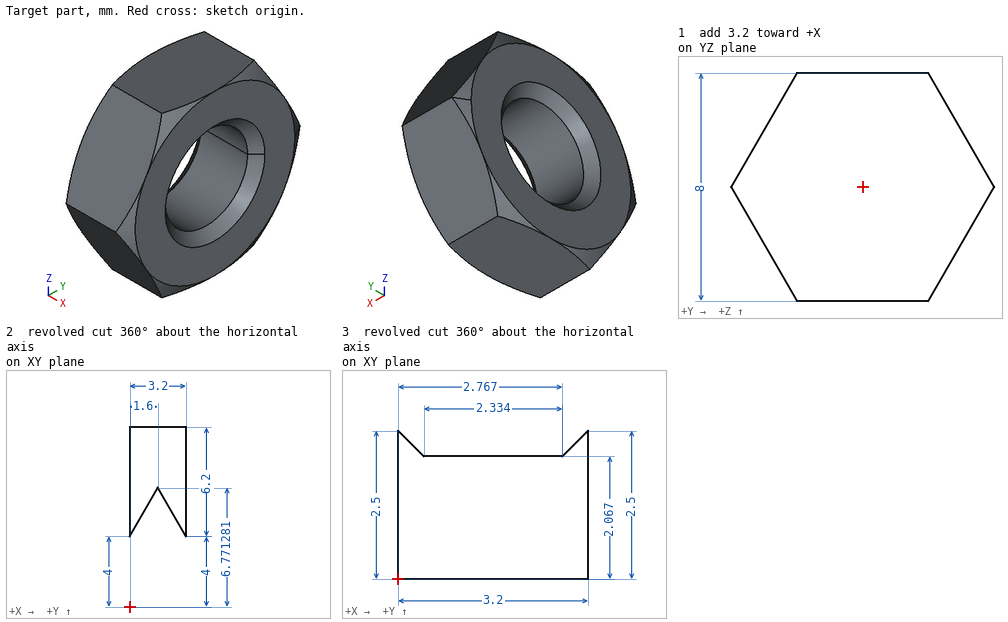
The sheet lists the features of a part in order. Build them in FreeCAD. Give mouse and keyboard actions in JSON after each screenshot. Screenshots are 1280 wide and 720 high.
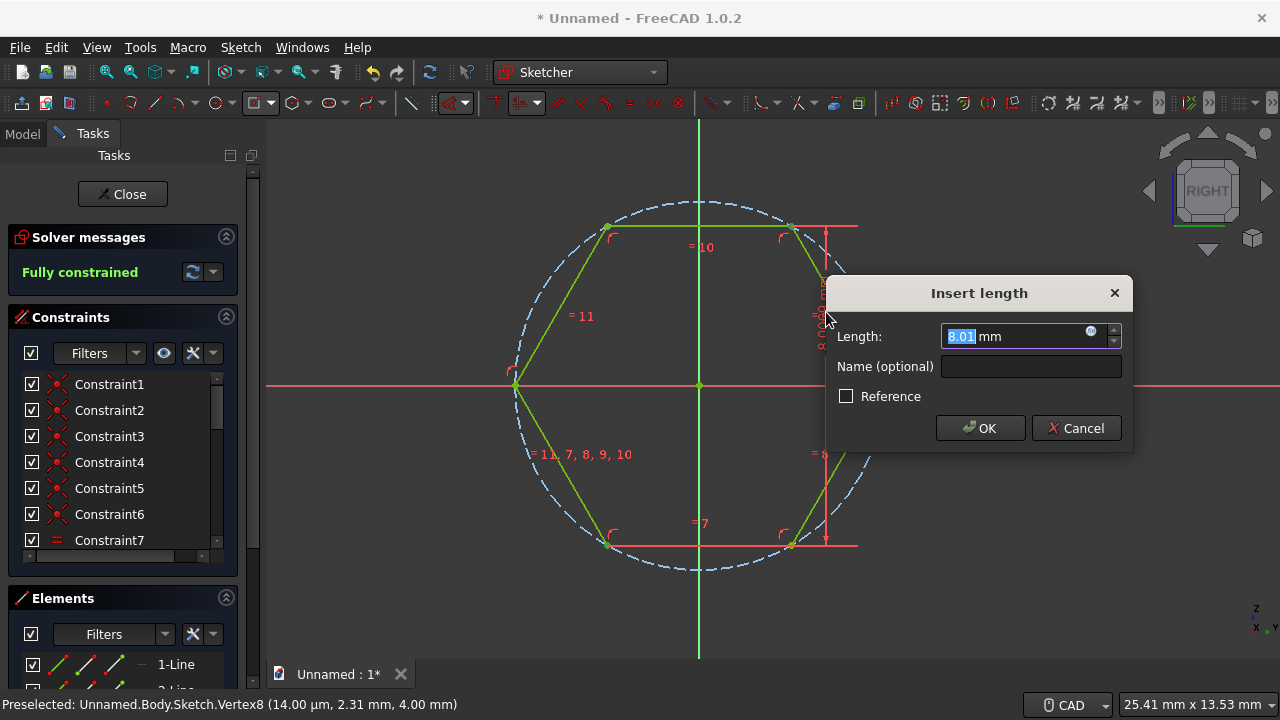
{"action": "type", "text": "8"}
{"action": "key", "text": "Return"}
{"action": "key", "text": "Escape"}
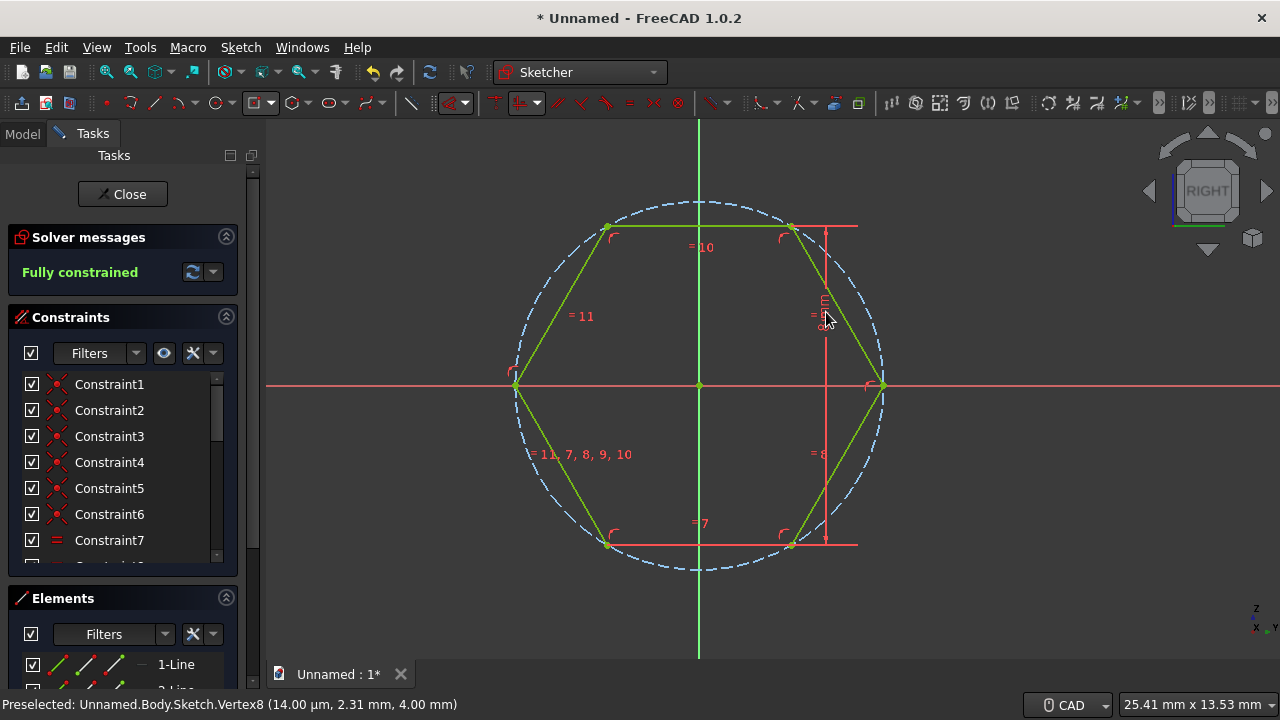
{"action": "left_click", "coordinate": [123, 194]}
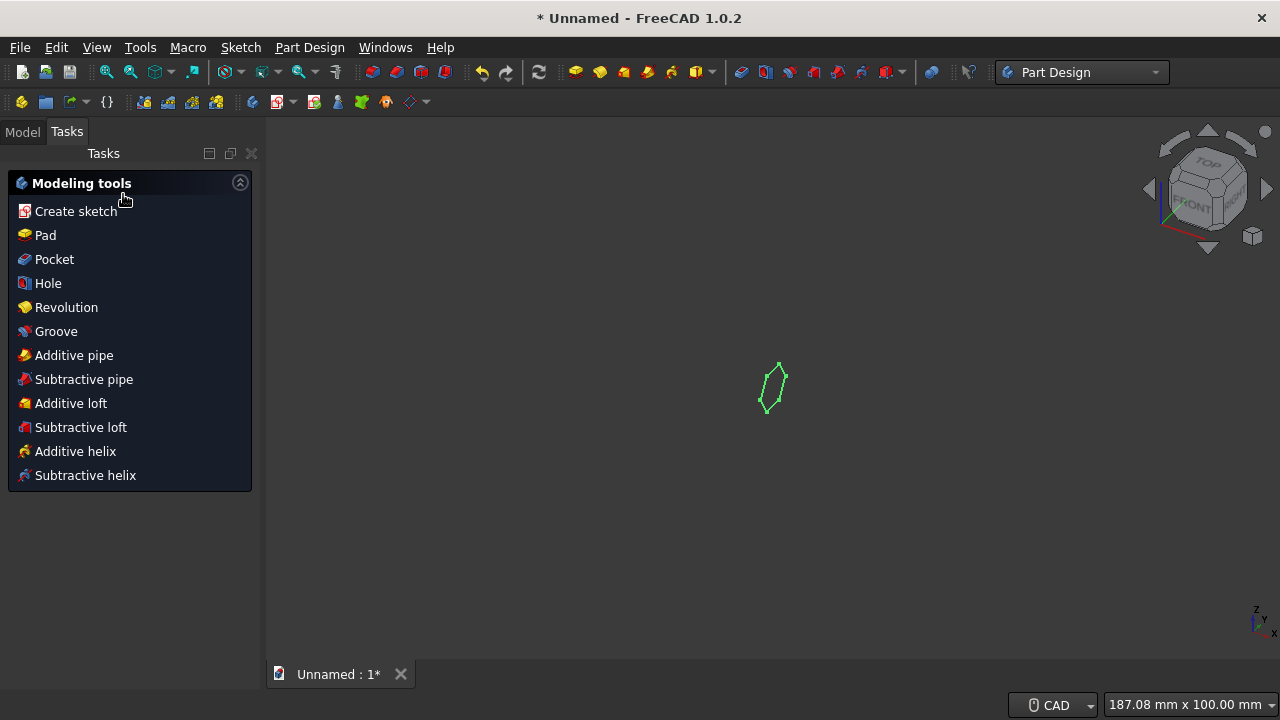
{"action": "left_click", "coordinate": [576, 72]}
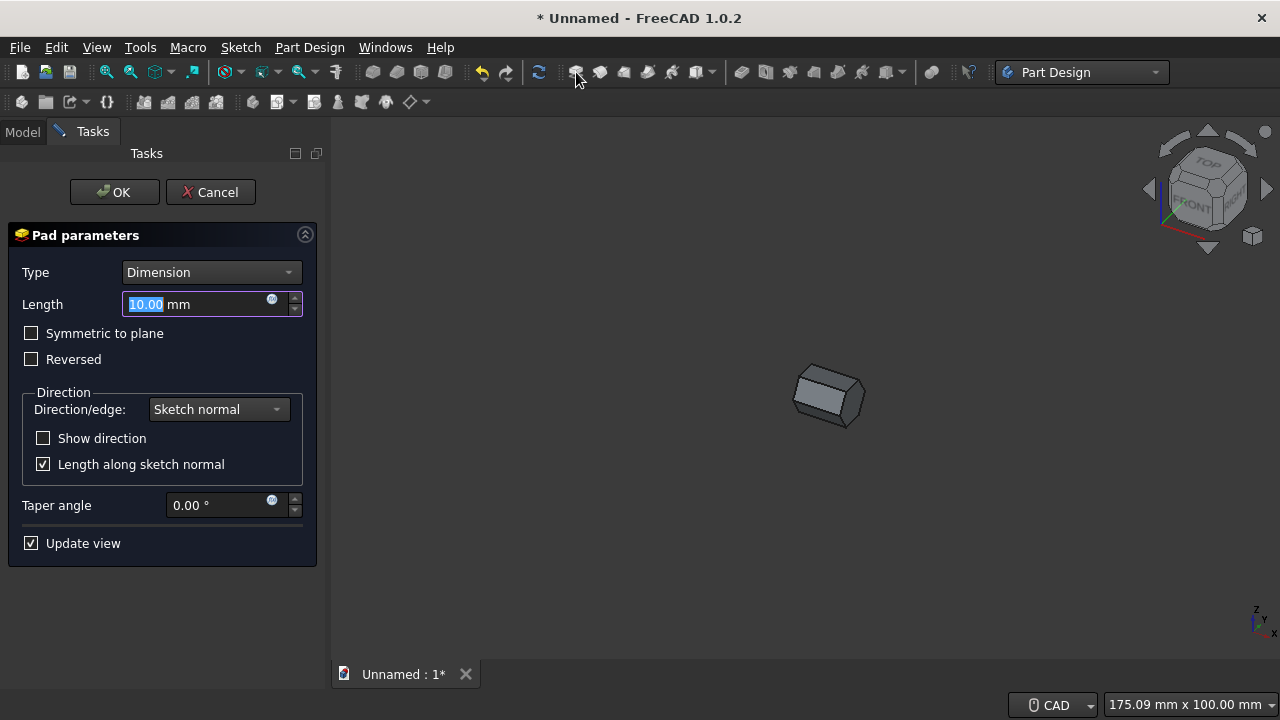
{"action": "type", "text": "3.2"}
{"action": "key", "text": "Tab"}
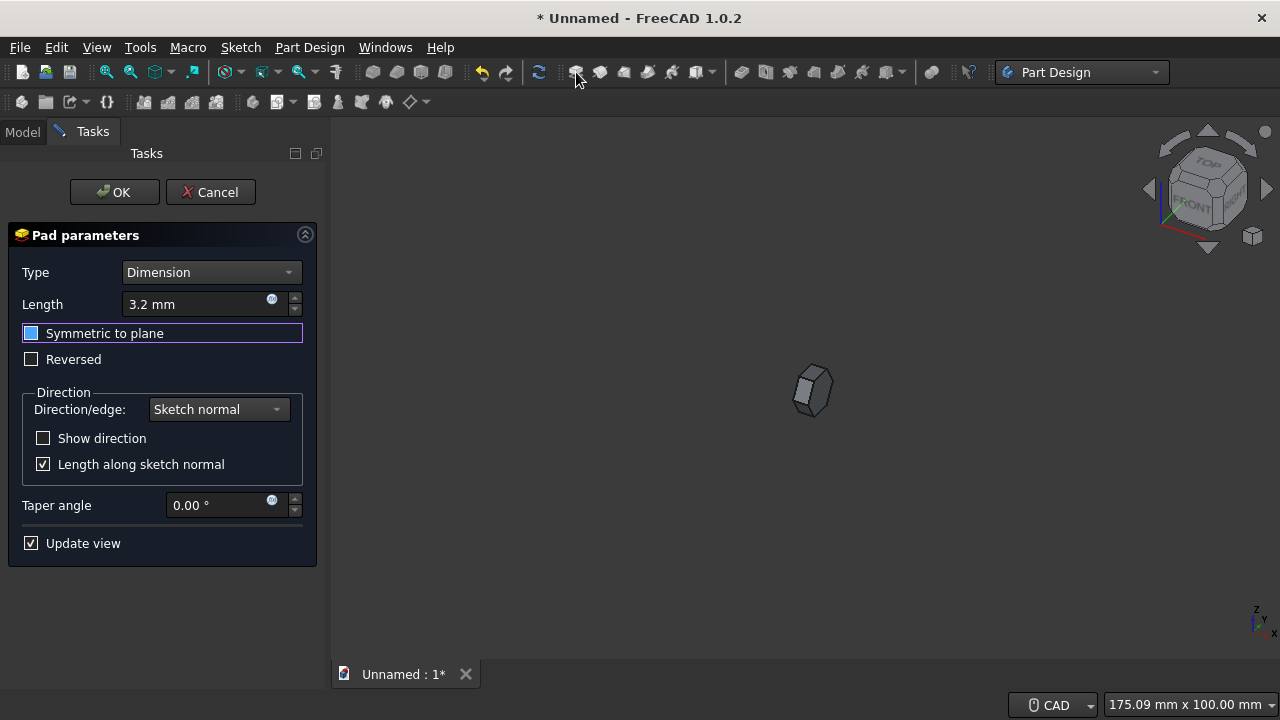
{"action": "left_click", "coordinate": [115, 192]}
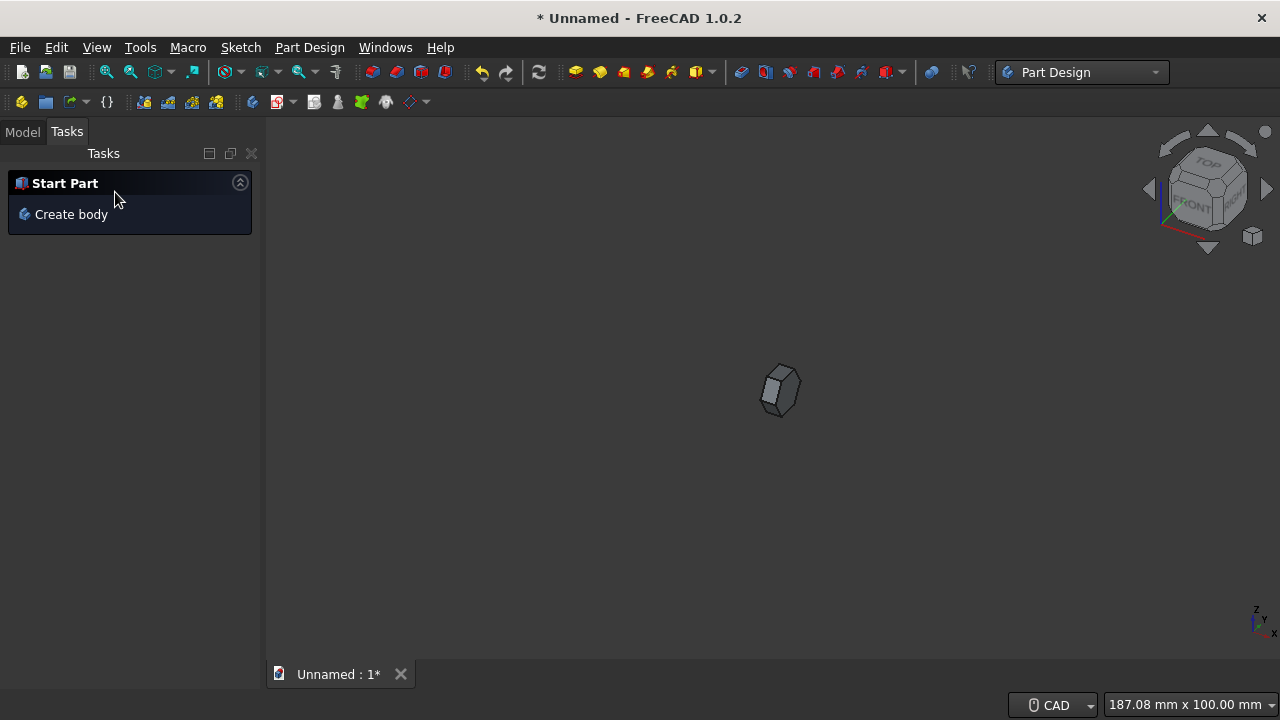
{"action": "left_click", "coordinate": [108, 72]}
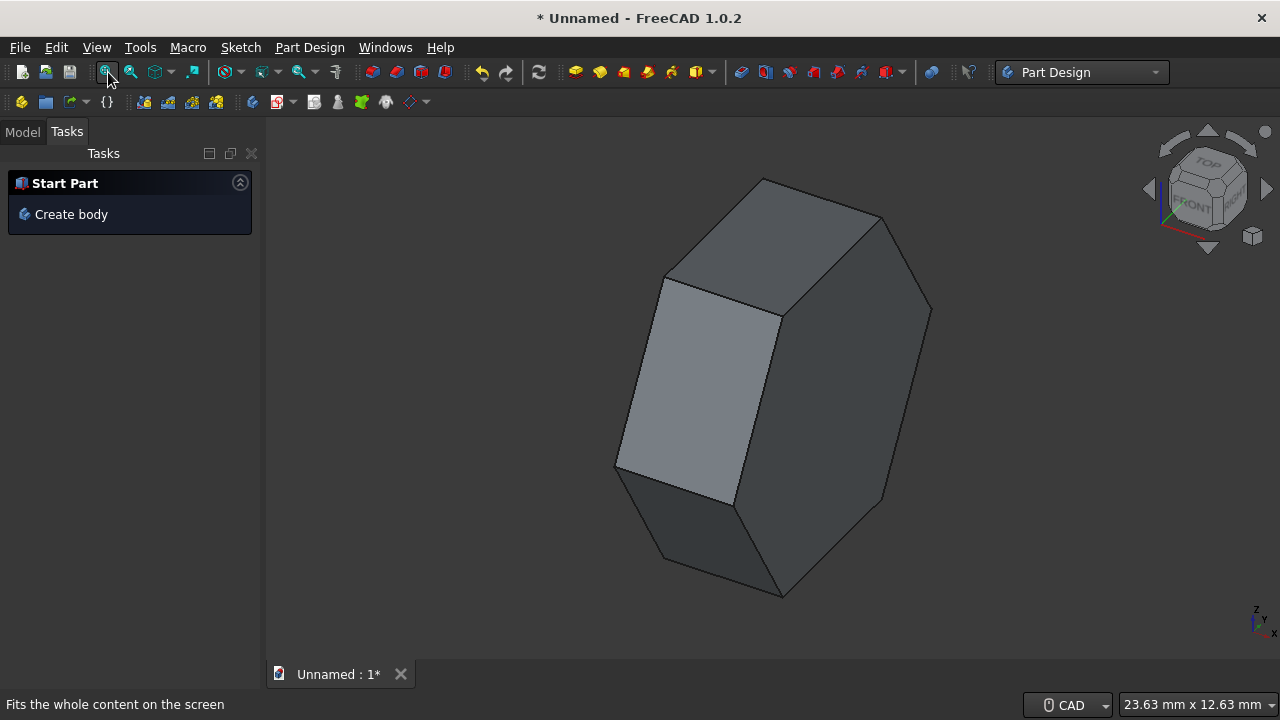
{"action": "left_click", "coordinate": [278, 102]}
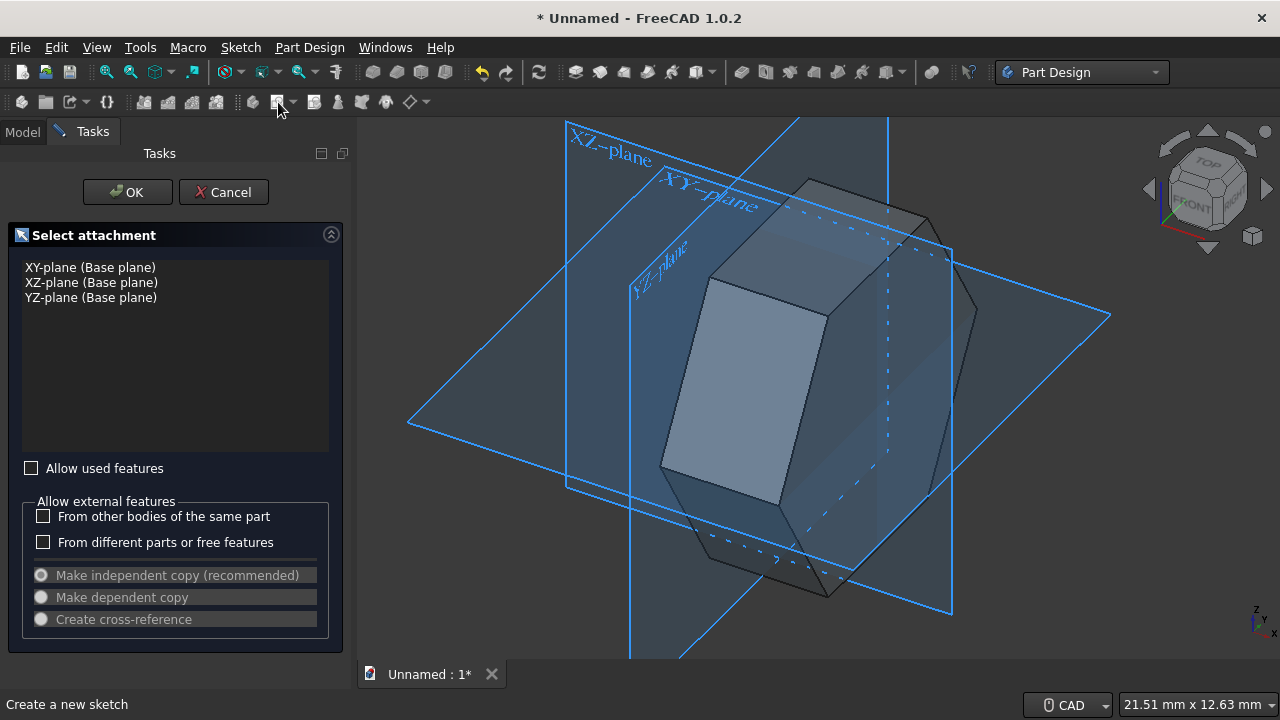
{"action": "left_click", "coordinate": [82, 268]}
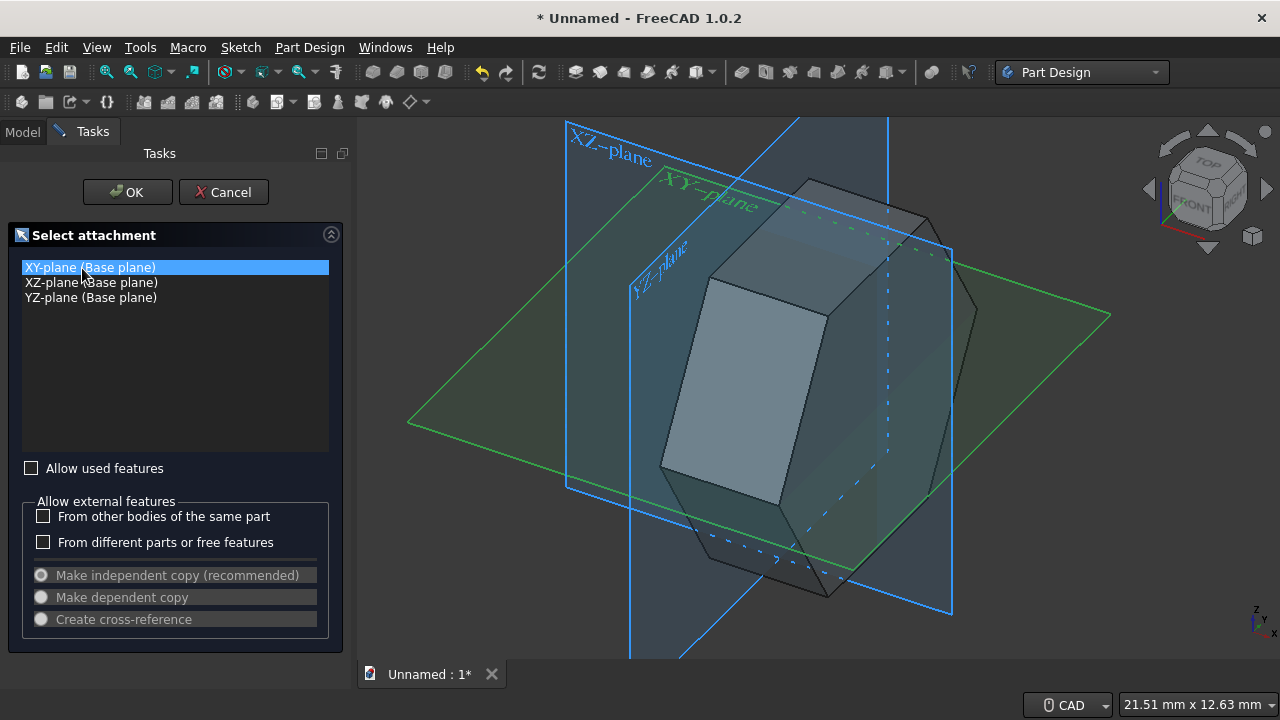
{"action": "left_click", "coordinate": [128, 192]}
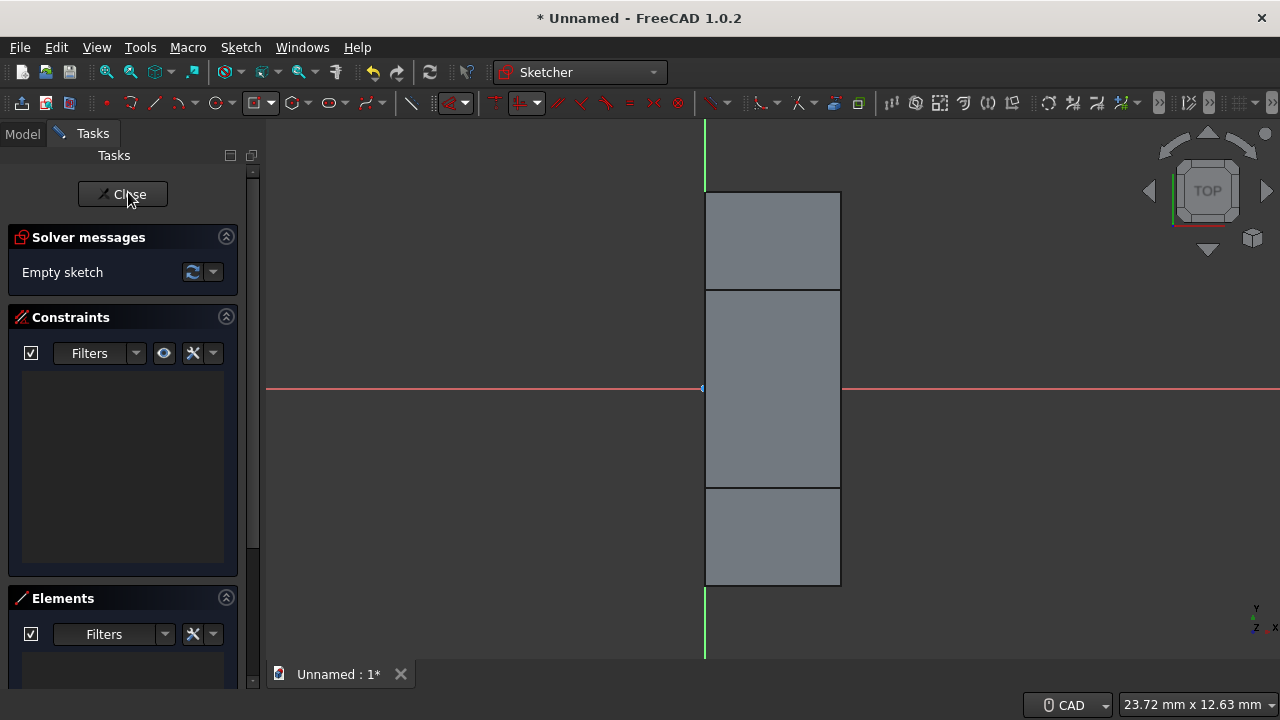
{"action": "key", "text": "q s"}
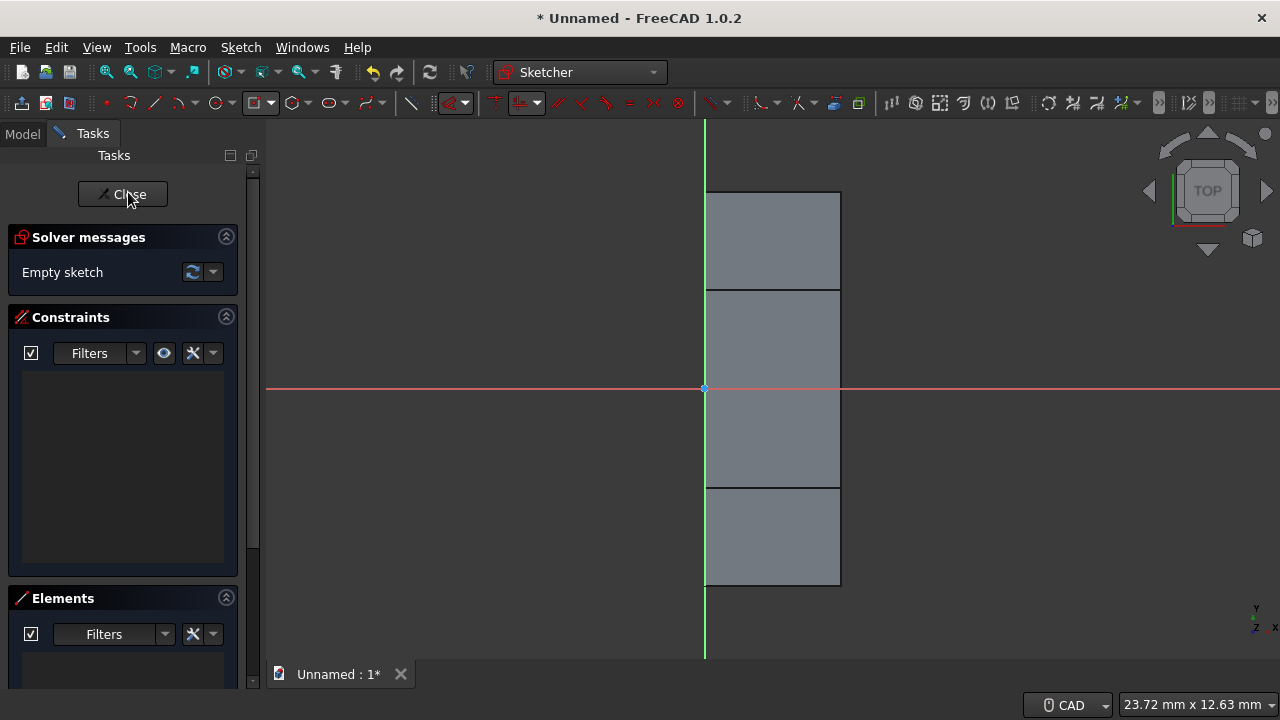
{"action": "scroll", "coordinate": [565, 631], "scroll_direction": "down", "scroll_amount": 2}